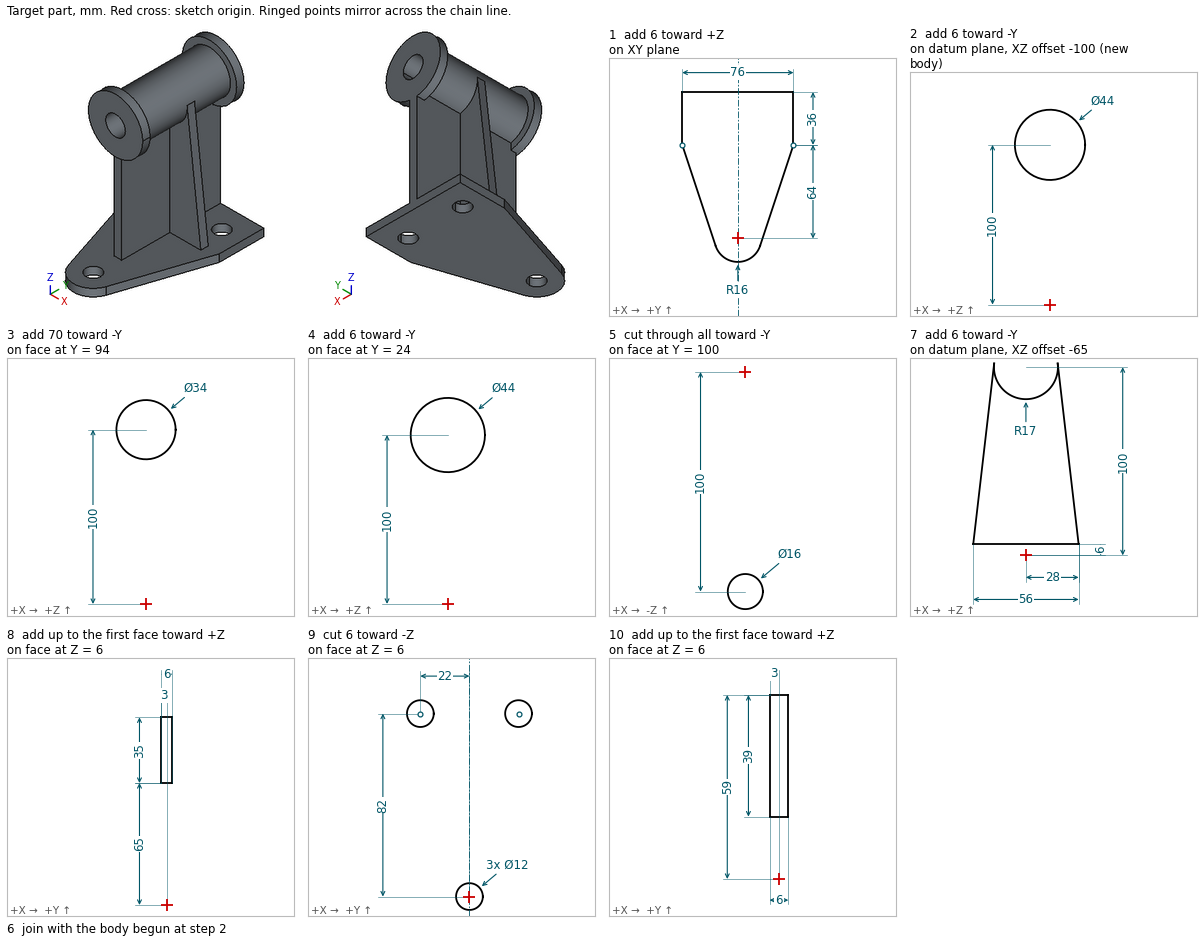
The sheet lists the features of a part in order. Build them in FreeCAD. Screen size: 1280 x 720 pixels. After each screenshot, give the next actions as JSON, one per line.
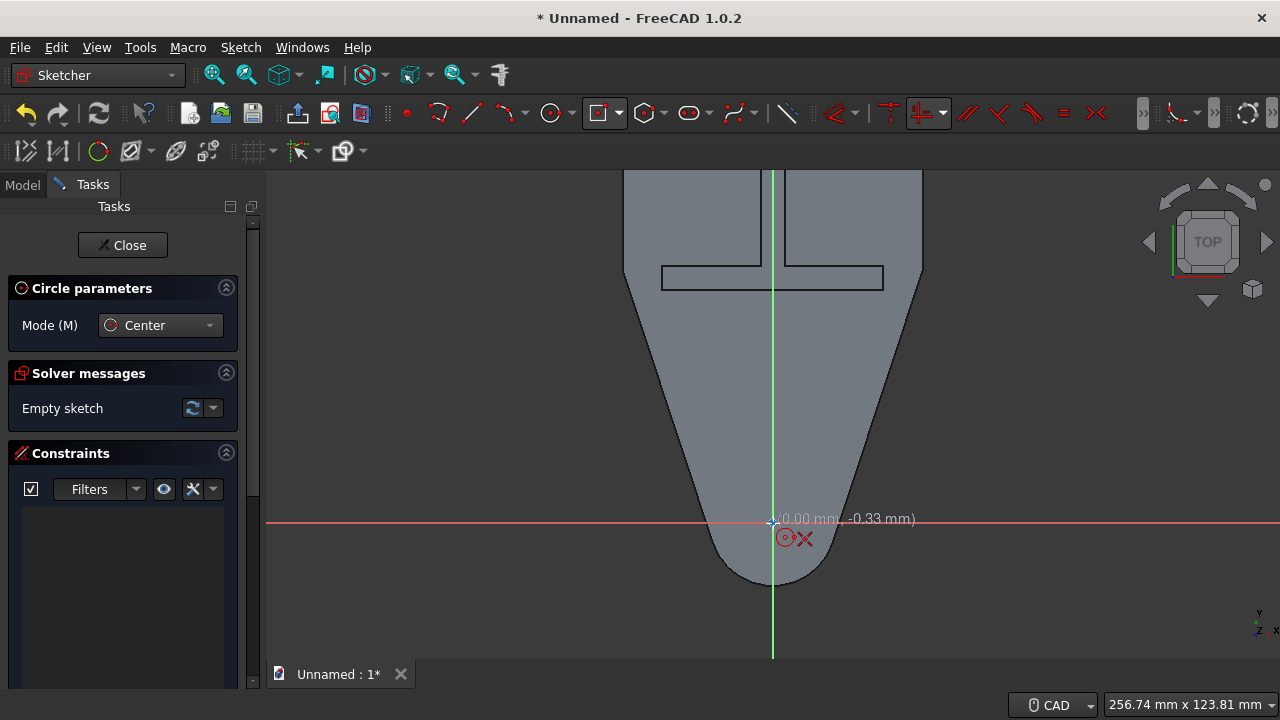
{"action": "left_click", "coordinate": [773, 523]}
{"action": "left_click", "coordinate": [790, 506]}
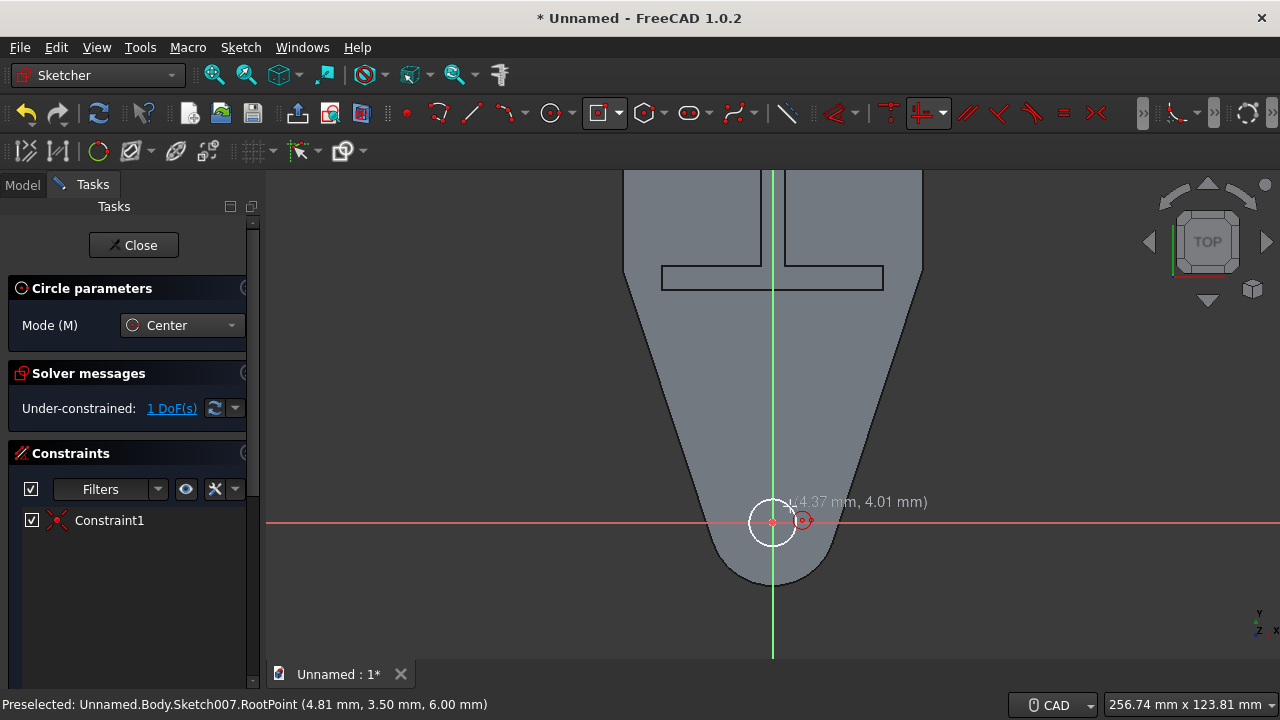
{"action": "left_click", "coordinate": [686, 199]}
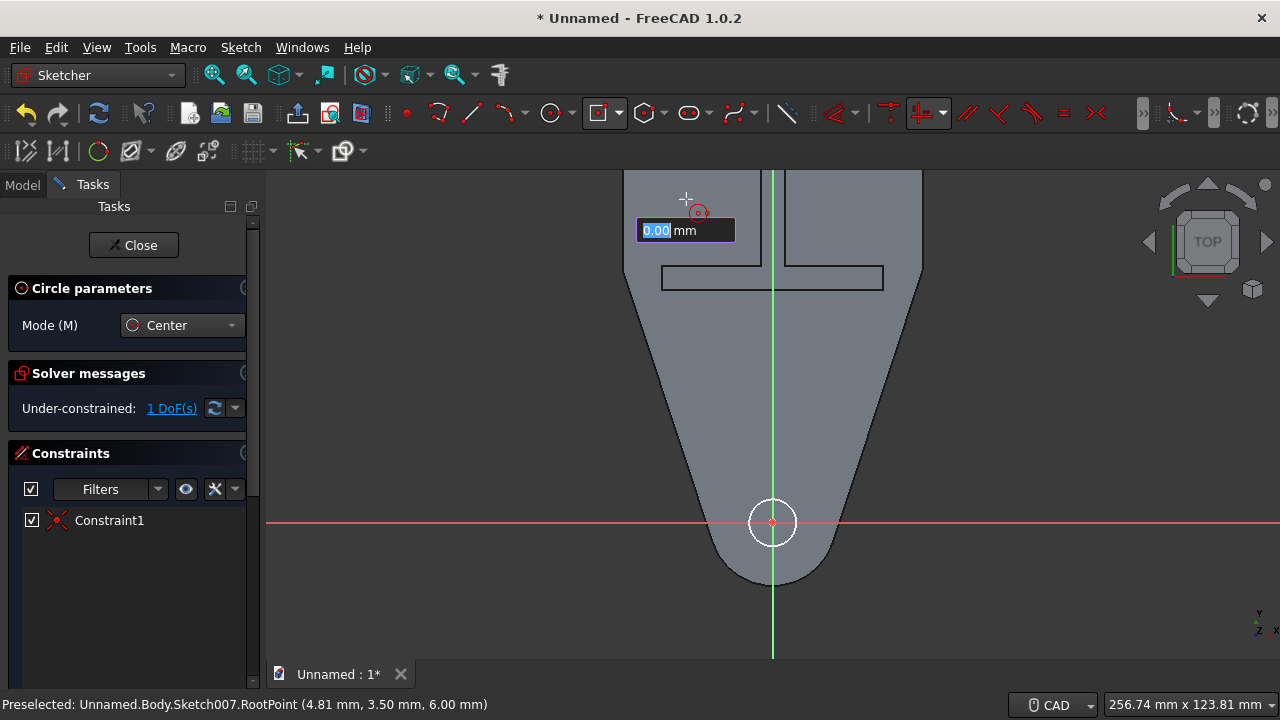
{"action": "scroll", "coordinate": [396, 631], "scroll_direction": "down", "scroll_amount": 1}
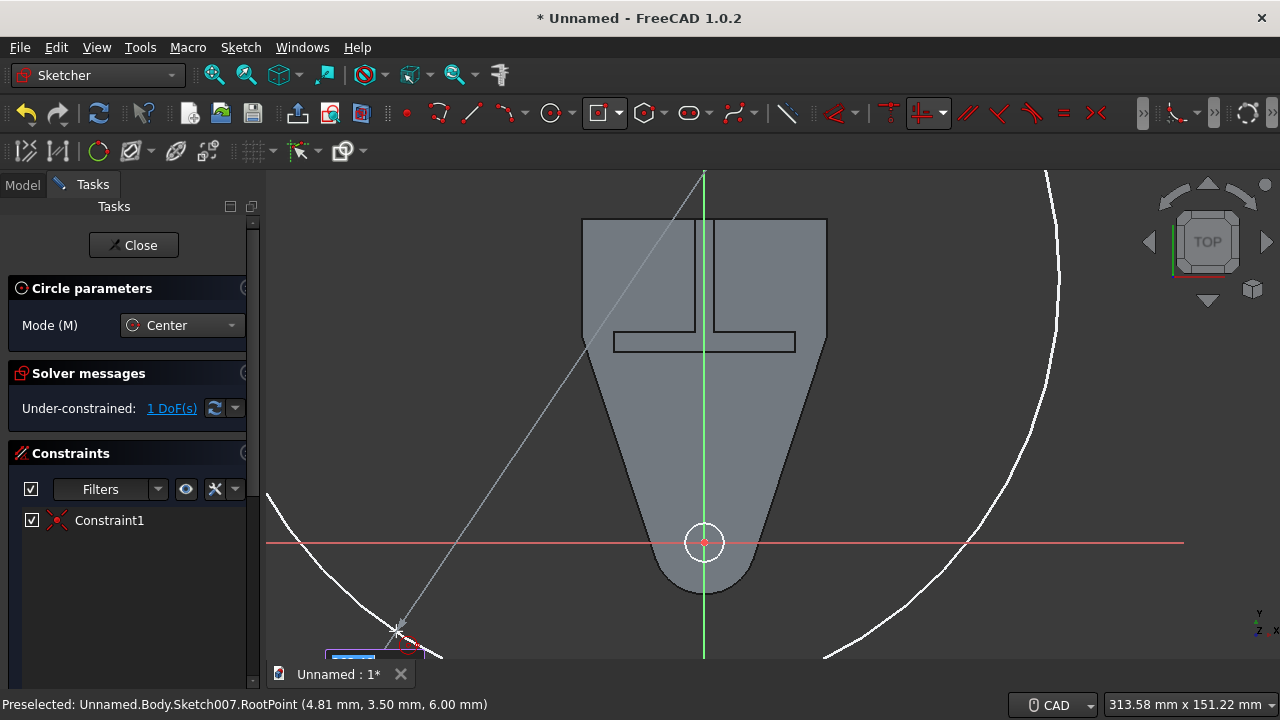
{"action": "left_click", "coordinate": [647, 264]}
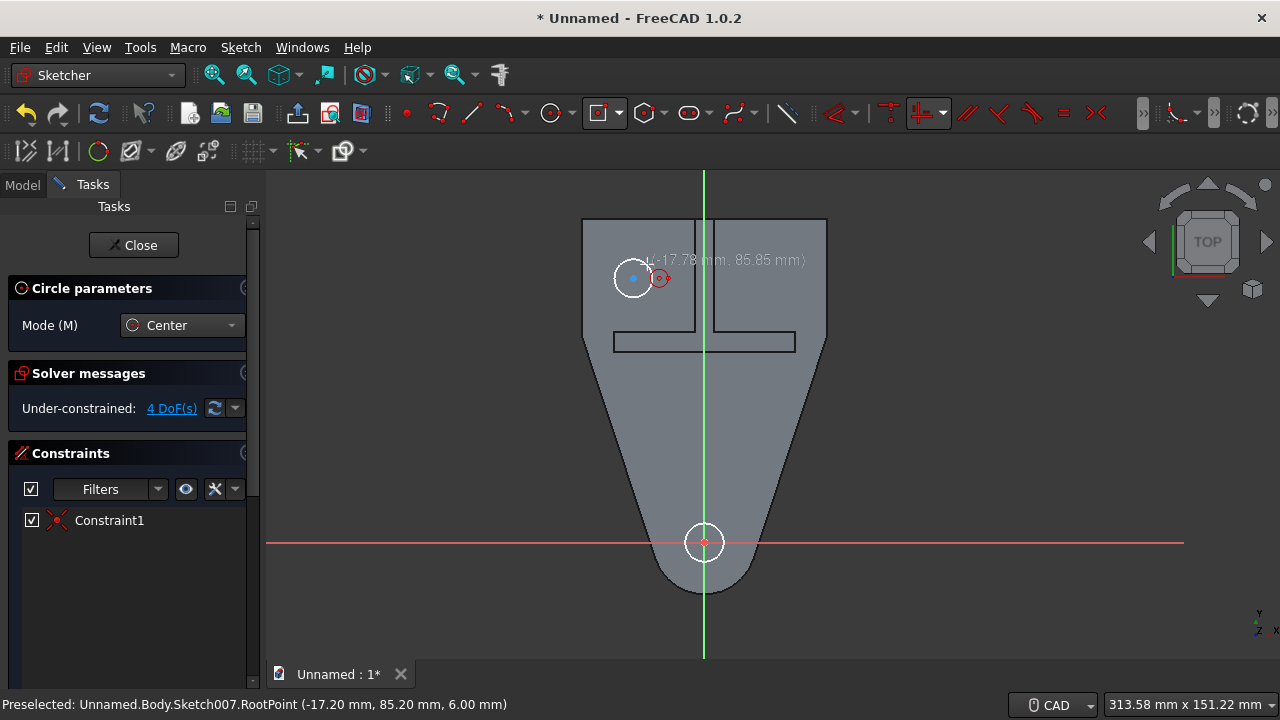
{"action": "left_click", "coordinate": [776, 277]}
{"action": "left_click", "coordinate": [789, 264]}
{"action": "key", "text": "Escape"}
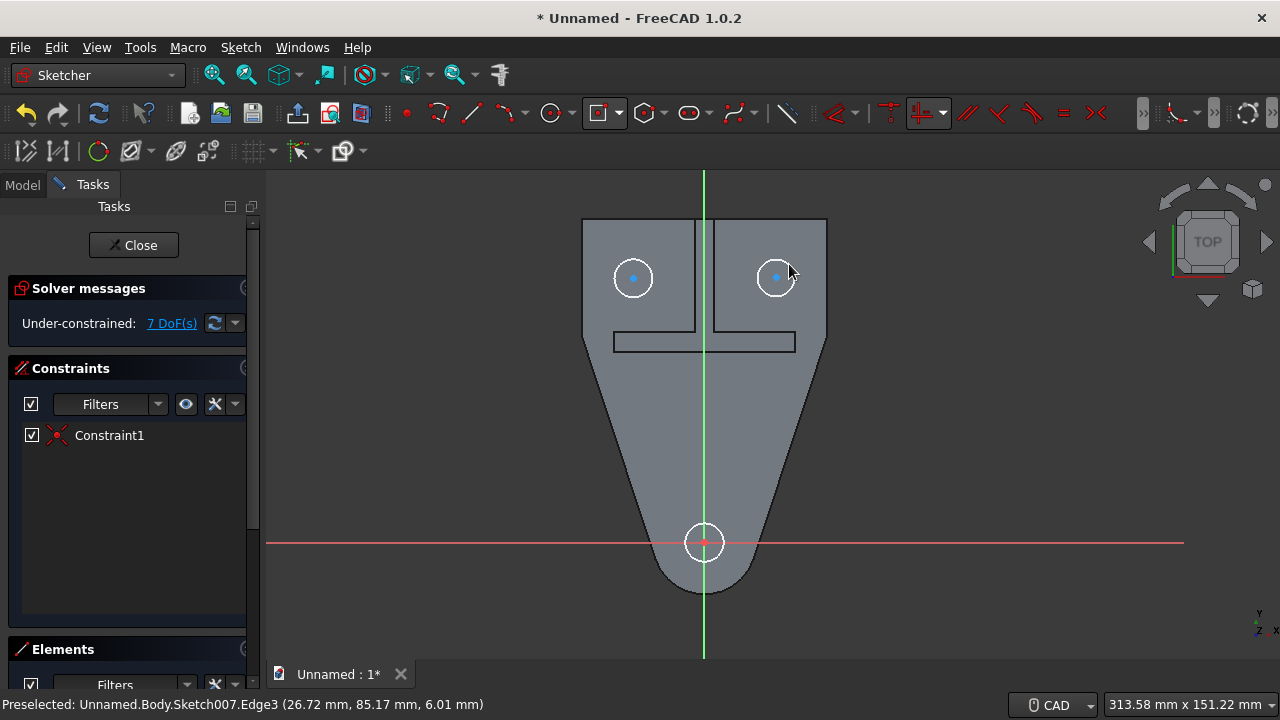
{"action": "left_click", "coordinate": [718, 529]}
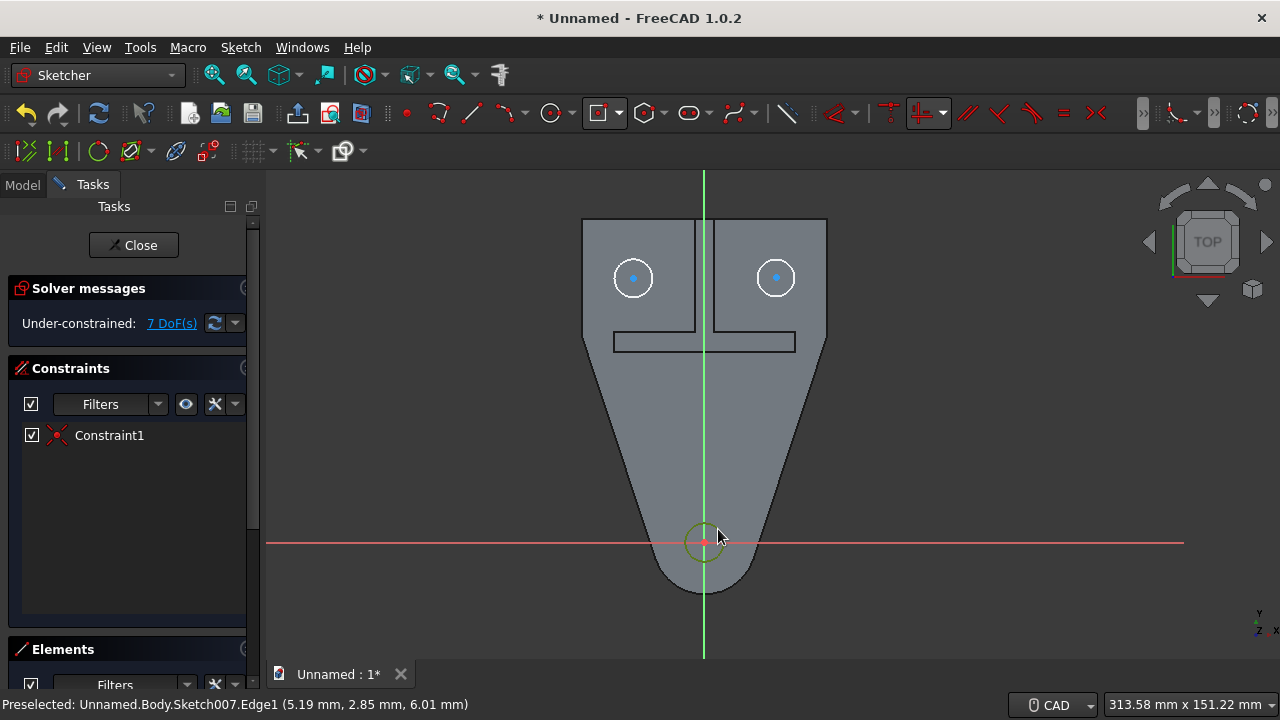
{"action": "left_click", "coordinate": [647, 265]}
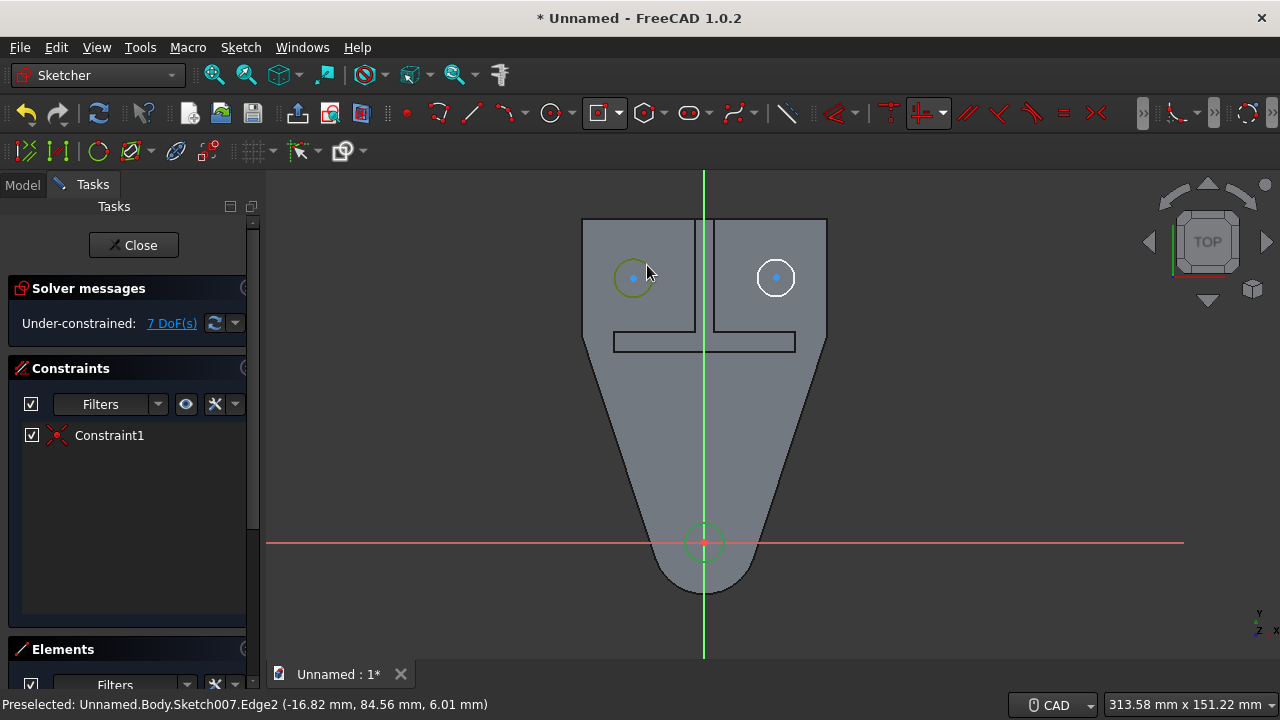
{"action": "left_click", "coordinate": [789, 265]}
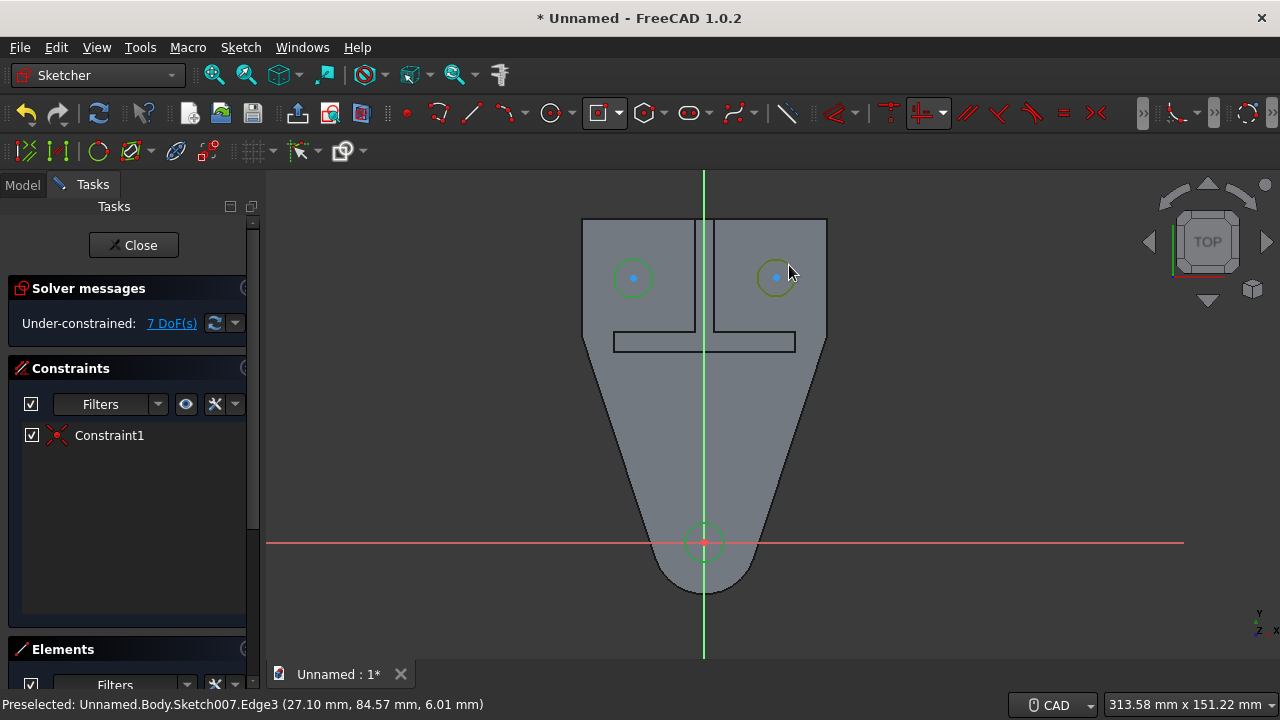
{"action": "left_click", "coordinate": [1064, 114]}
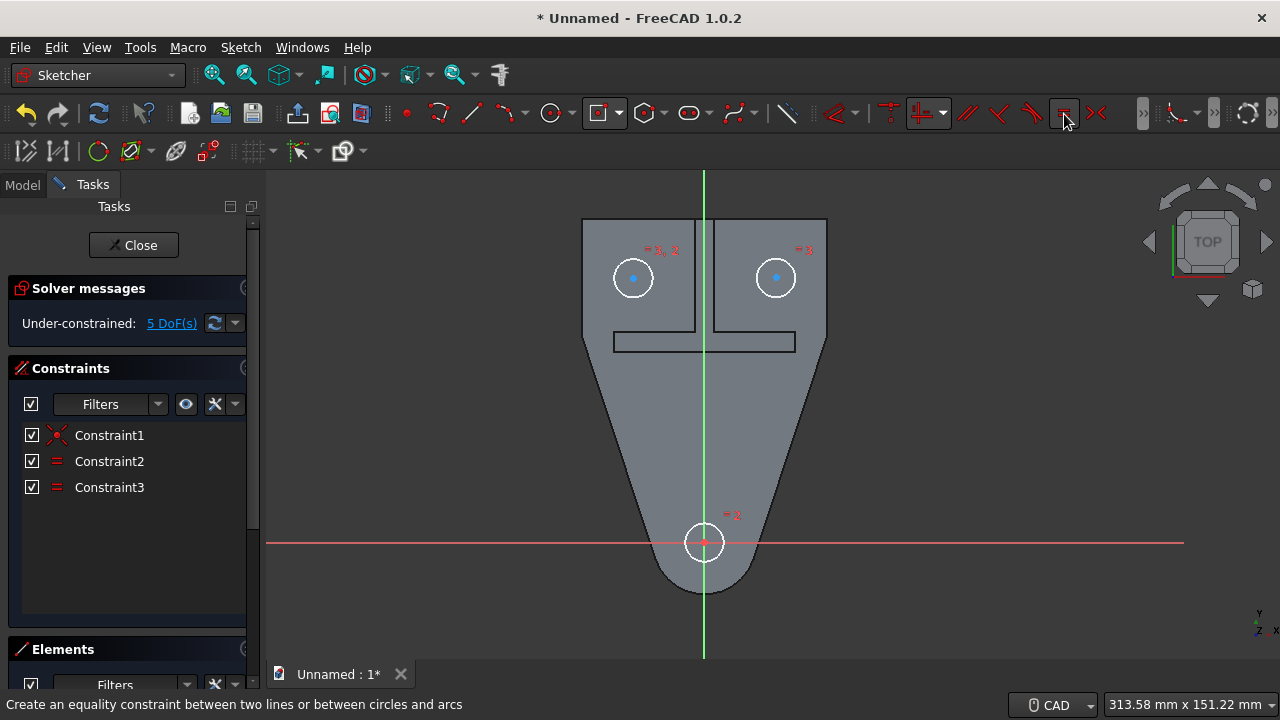
{"action": "left_click", "coordinate": [633, 278]}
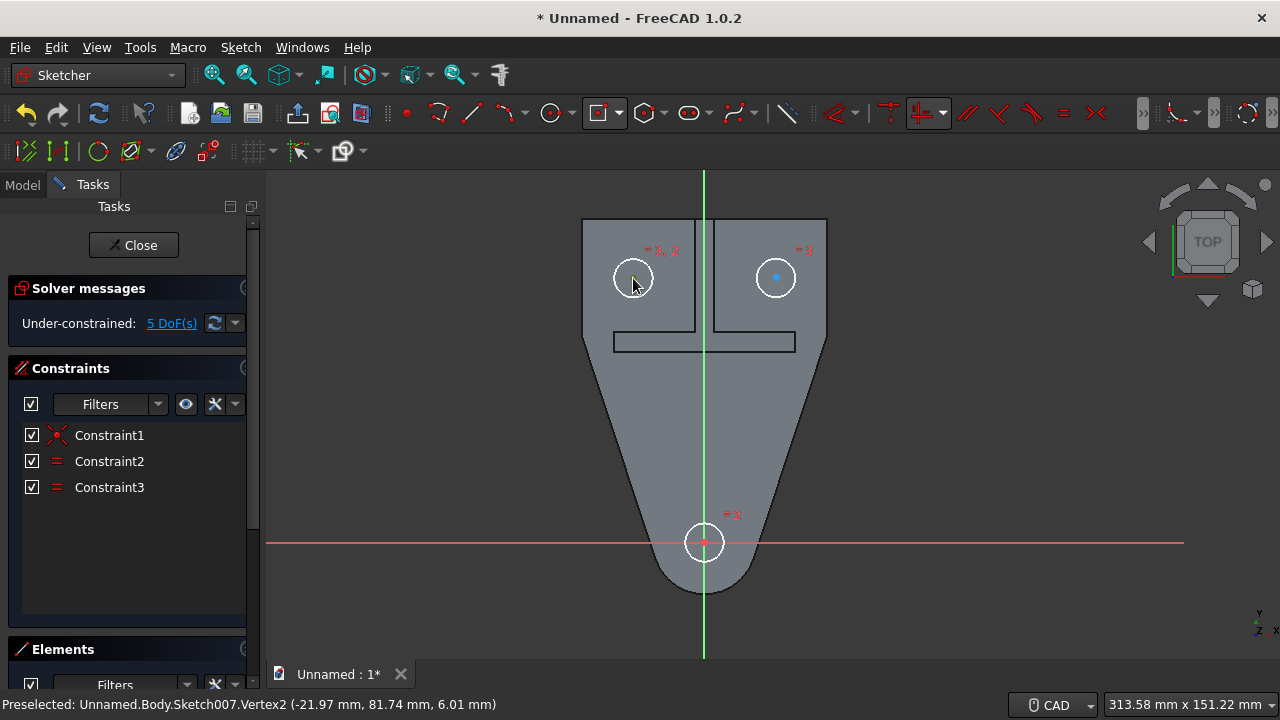
{"action": "left_click", "coordinate": [776, 278]}